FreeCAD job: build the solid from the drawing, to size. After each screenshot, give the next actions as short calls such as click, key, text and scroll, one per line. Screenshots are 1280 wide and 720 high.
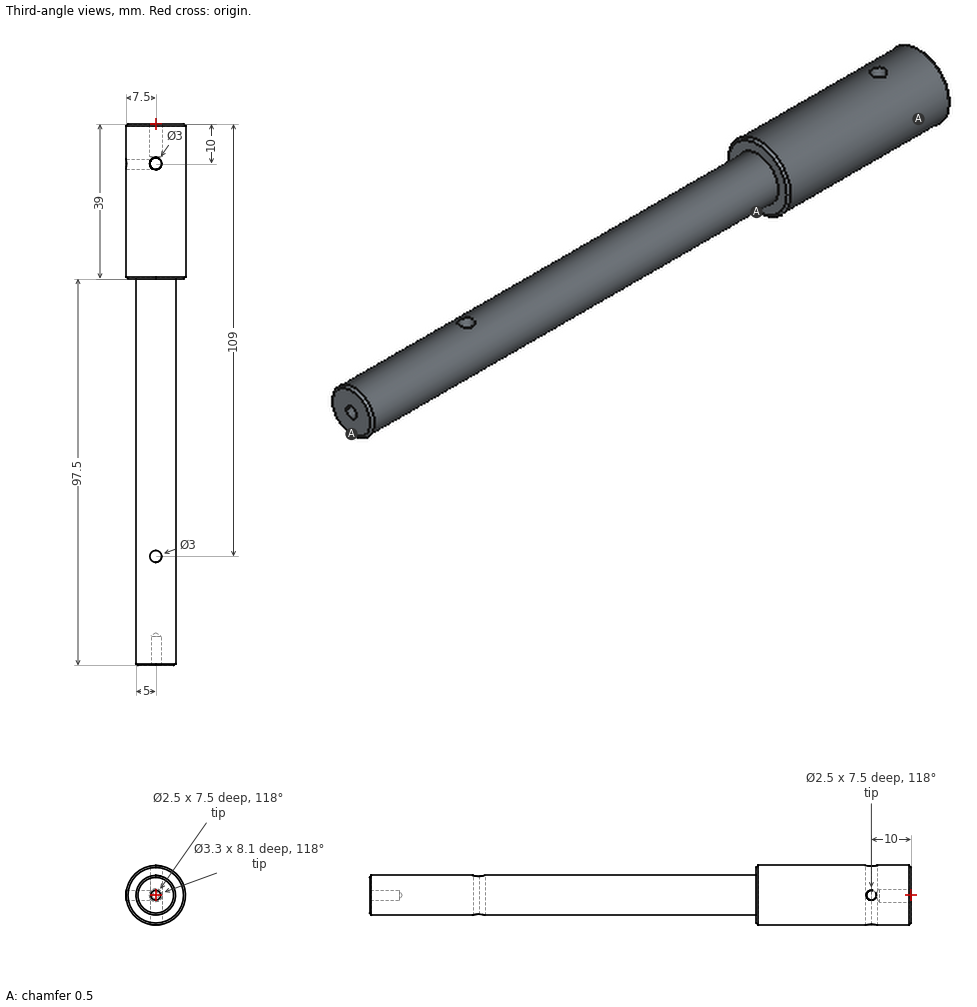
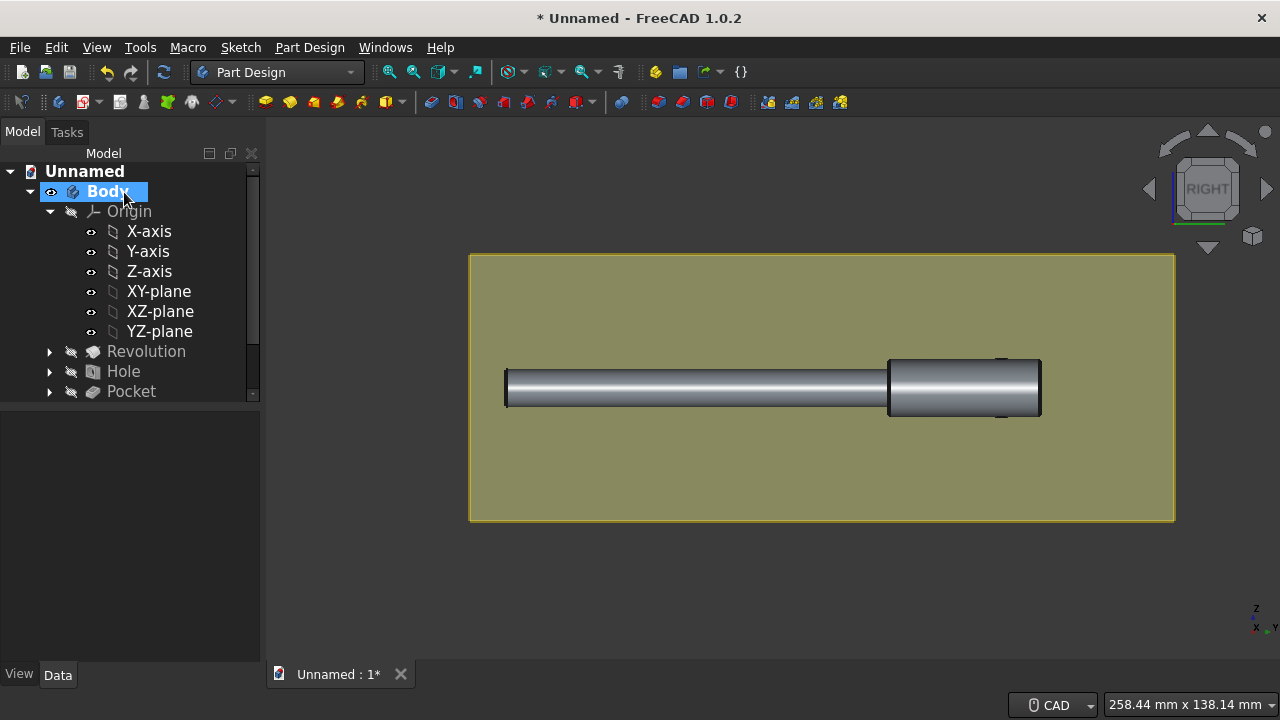
scroll(100, 287, down, 3)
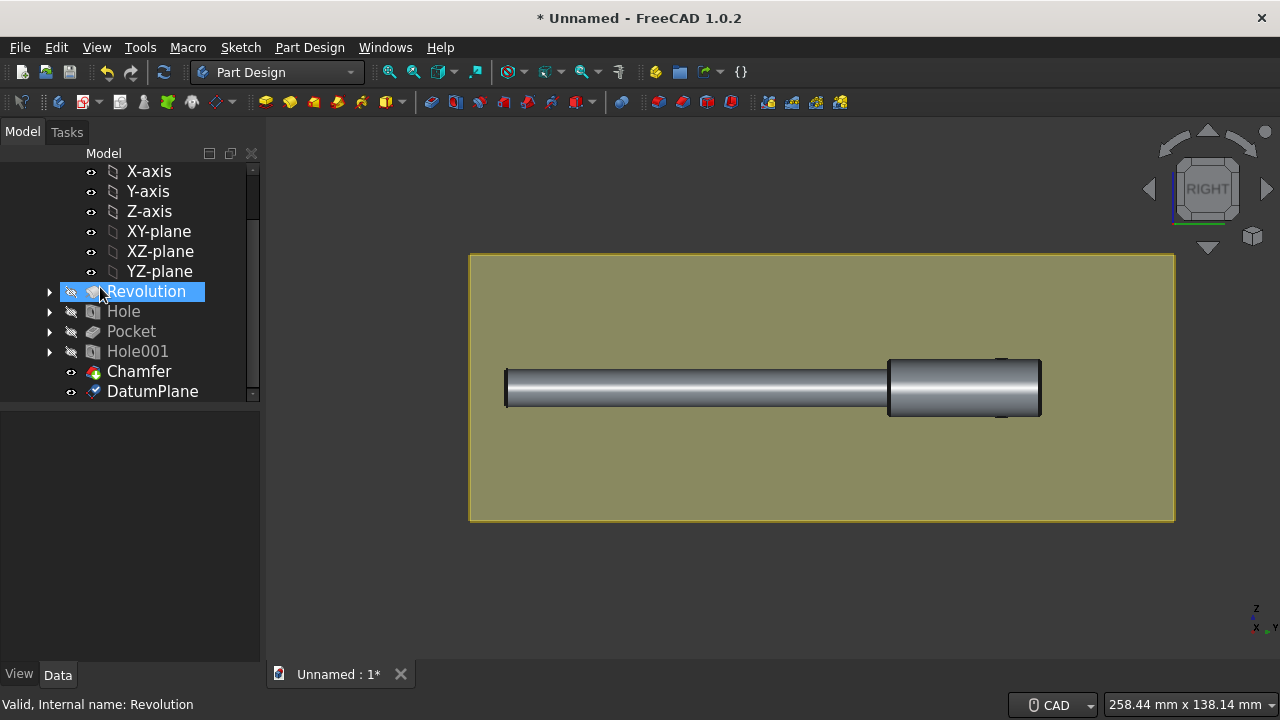
click(116, 392)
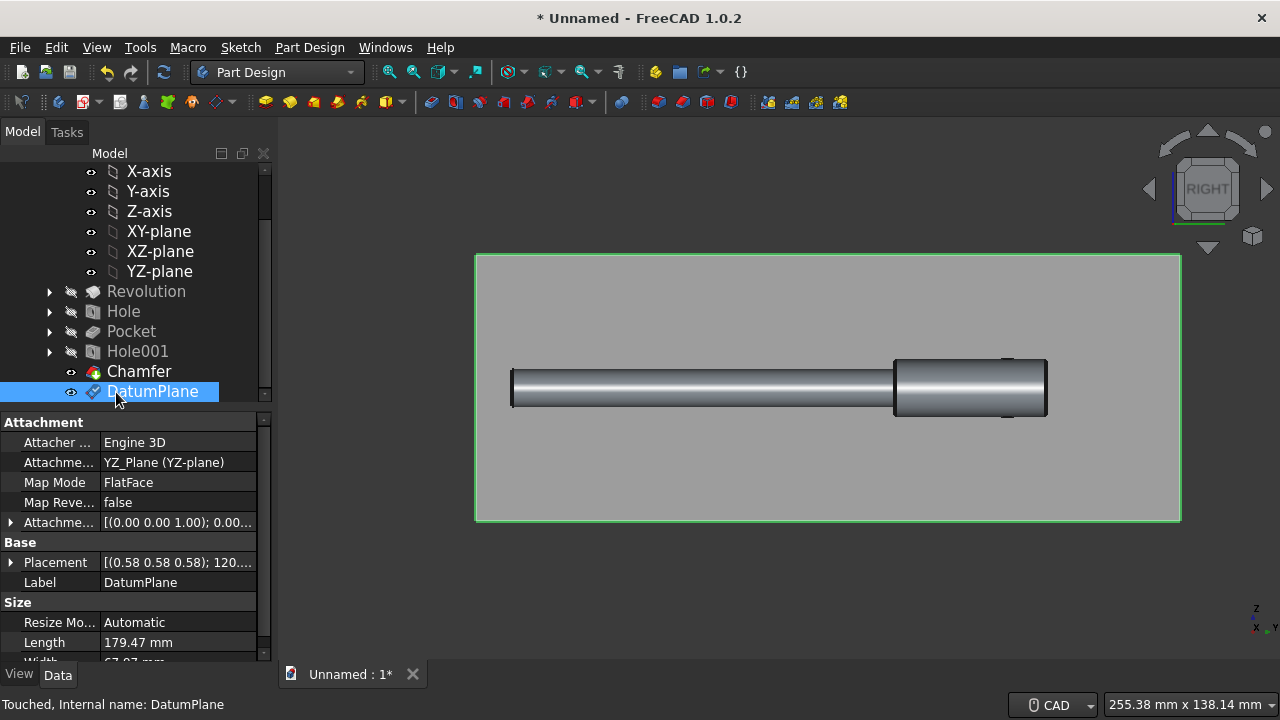
click(84, 102)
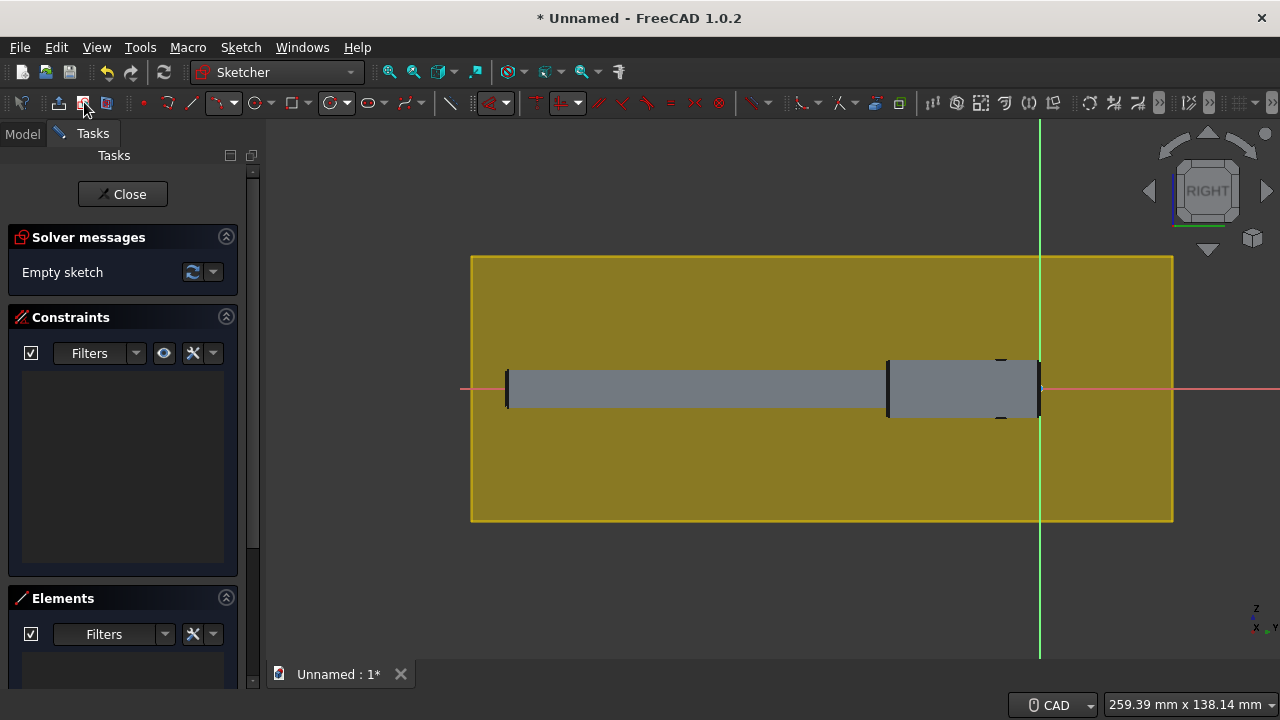
click(108, 104)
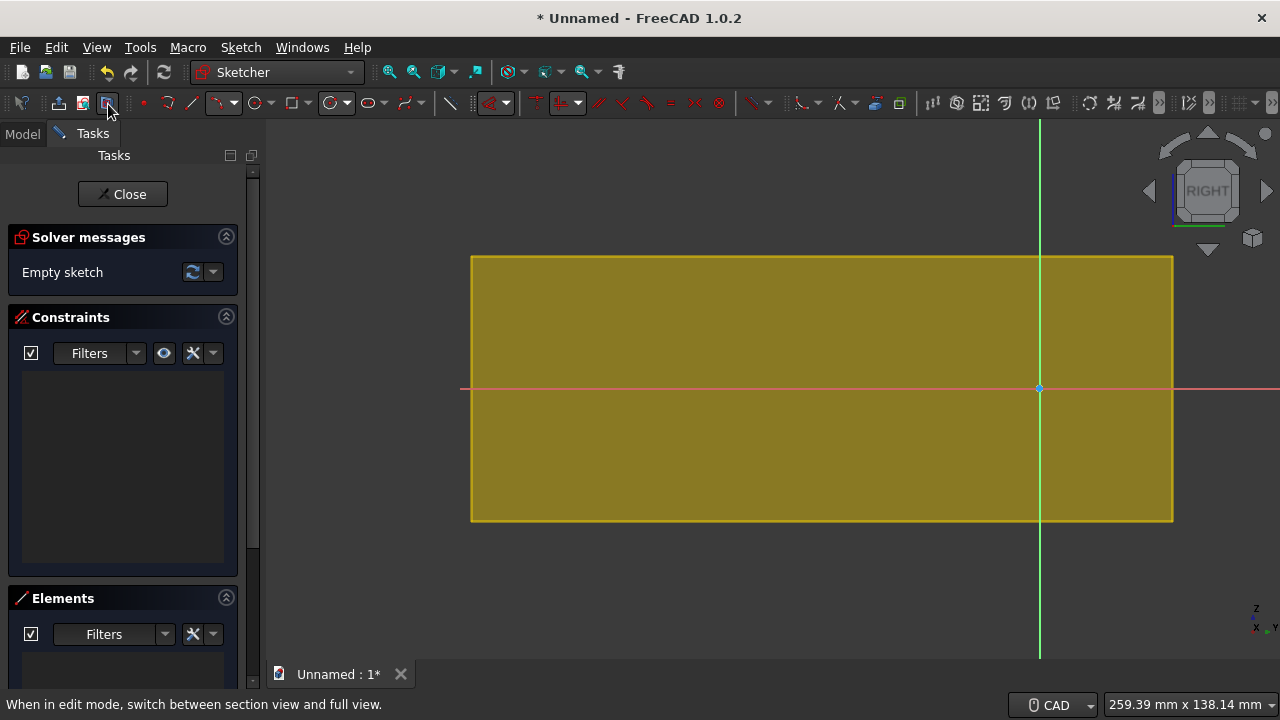
scroll(1016, 389, up, 15)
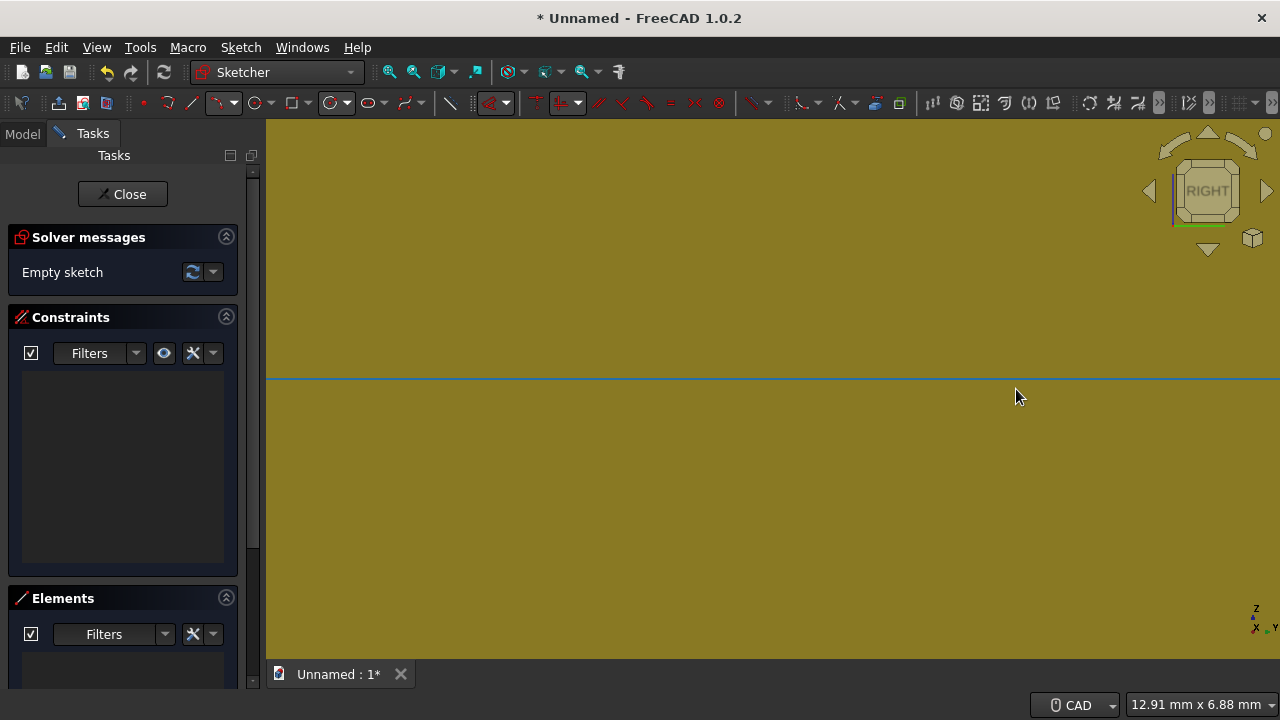
scroll(683, 368, up, 3)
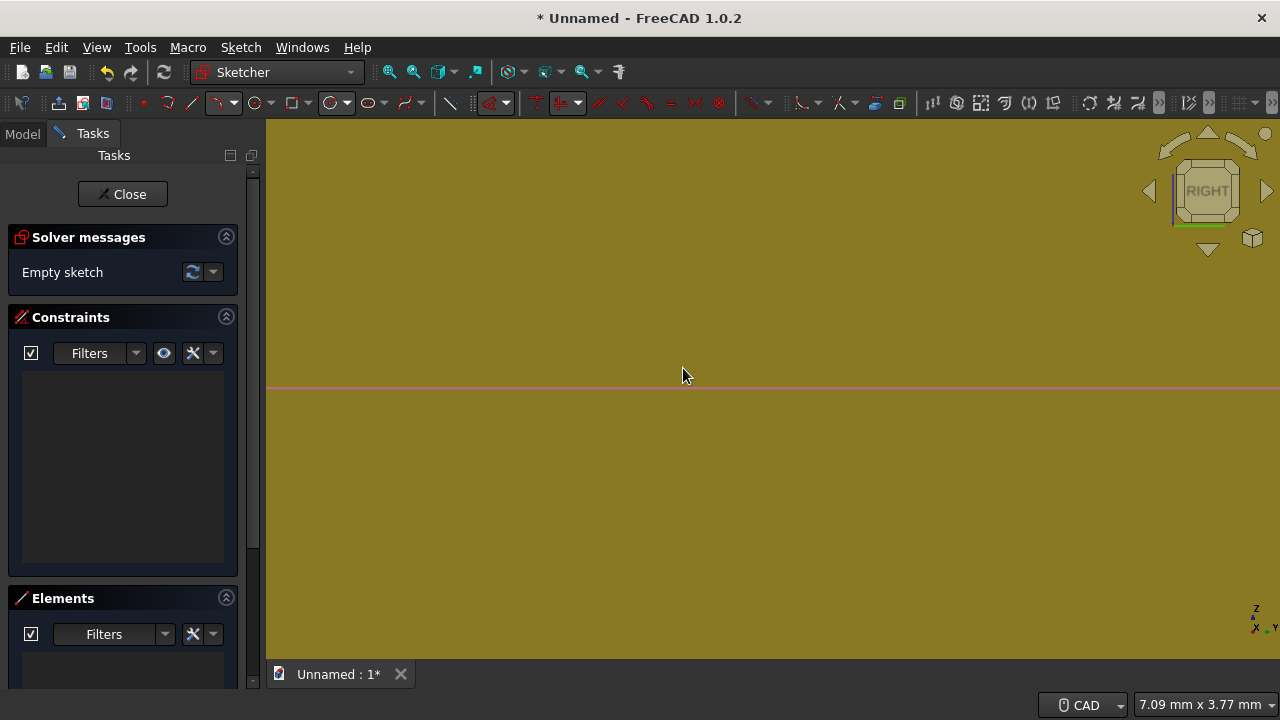
click(256, 104)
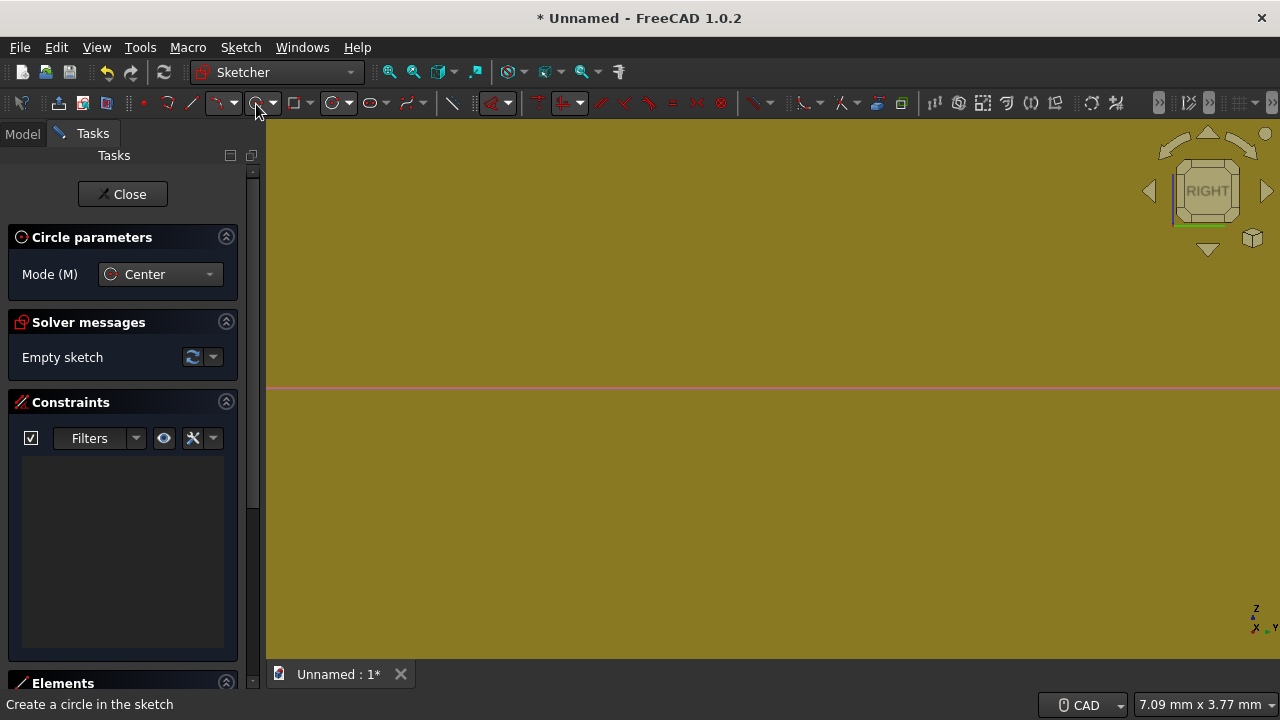
click(704, 388)
click(830, 262)
key(Escape)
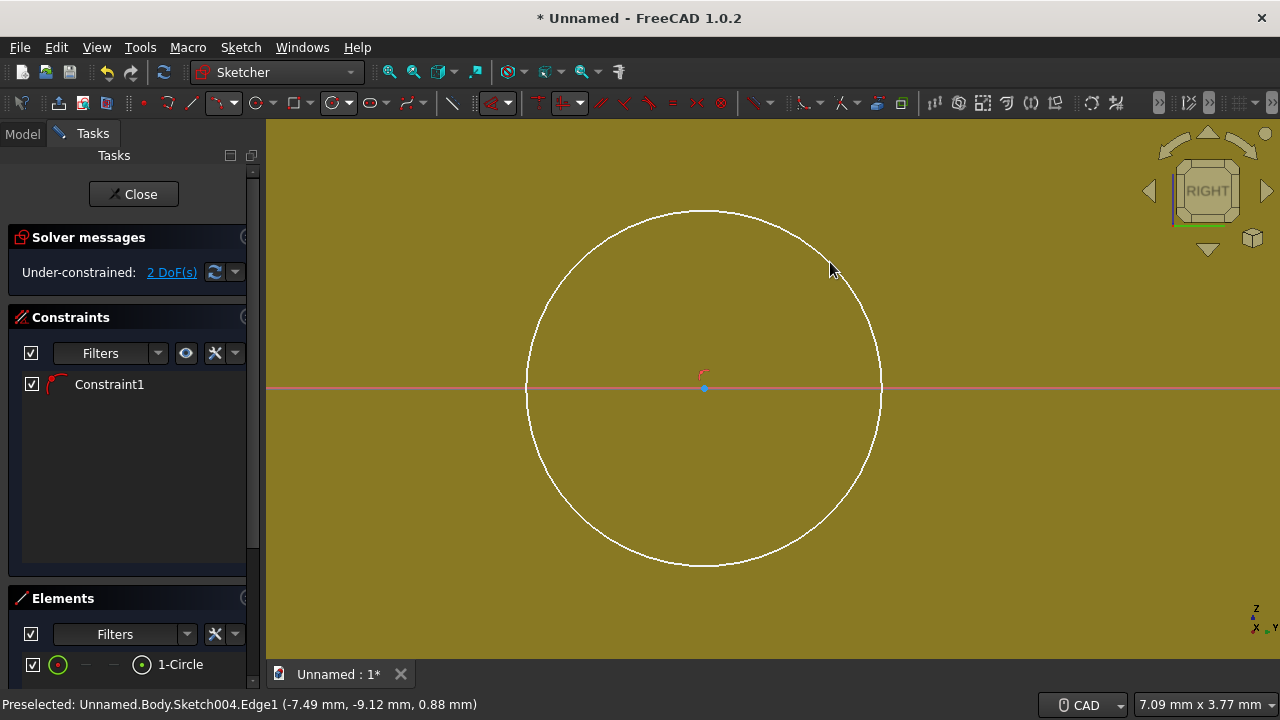
click(829, 262)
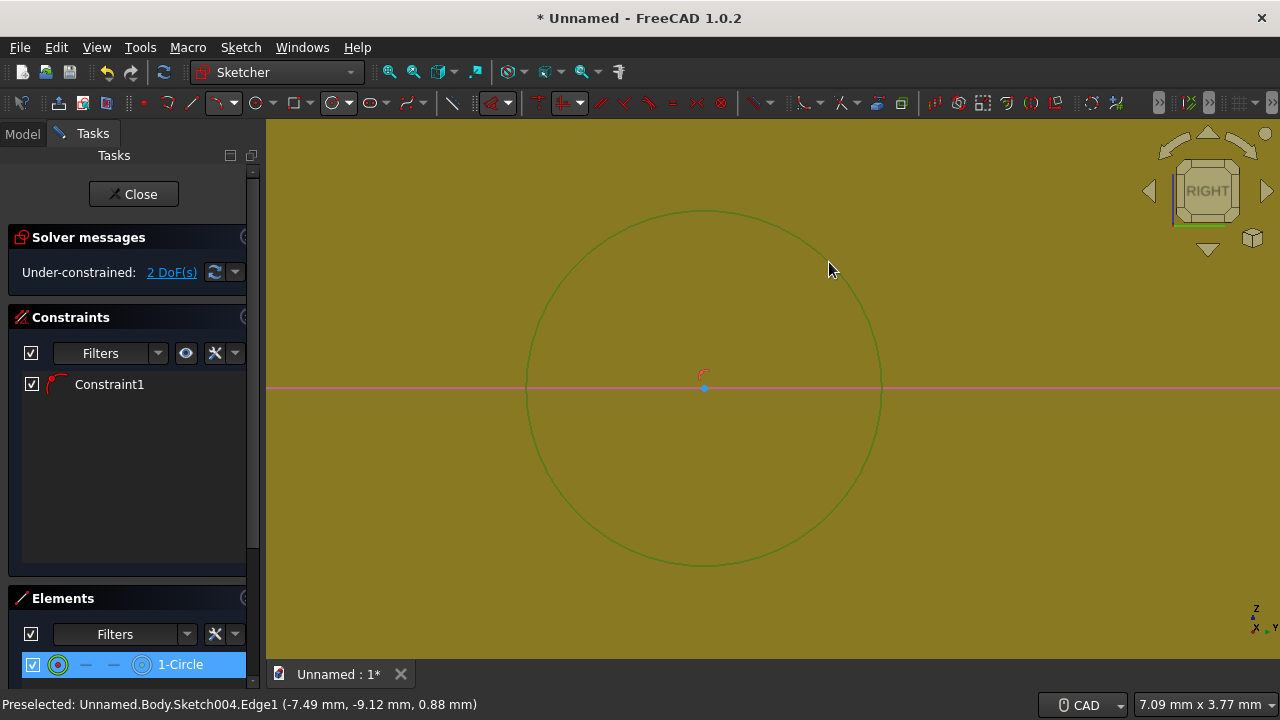
click(510, 104)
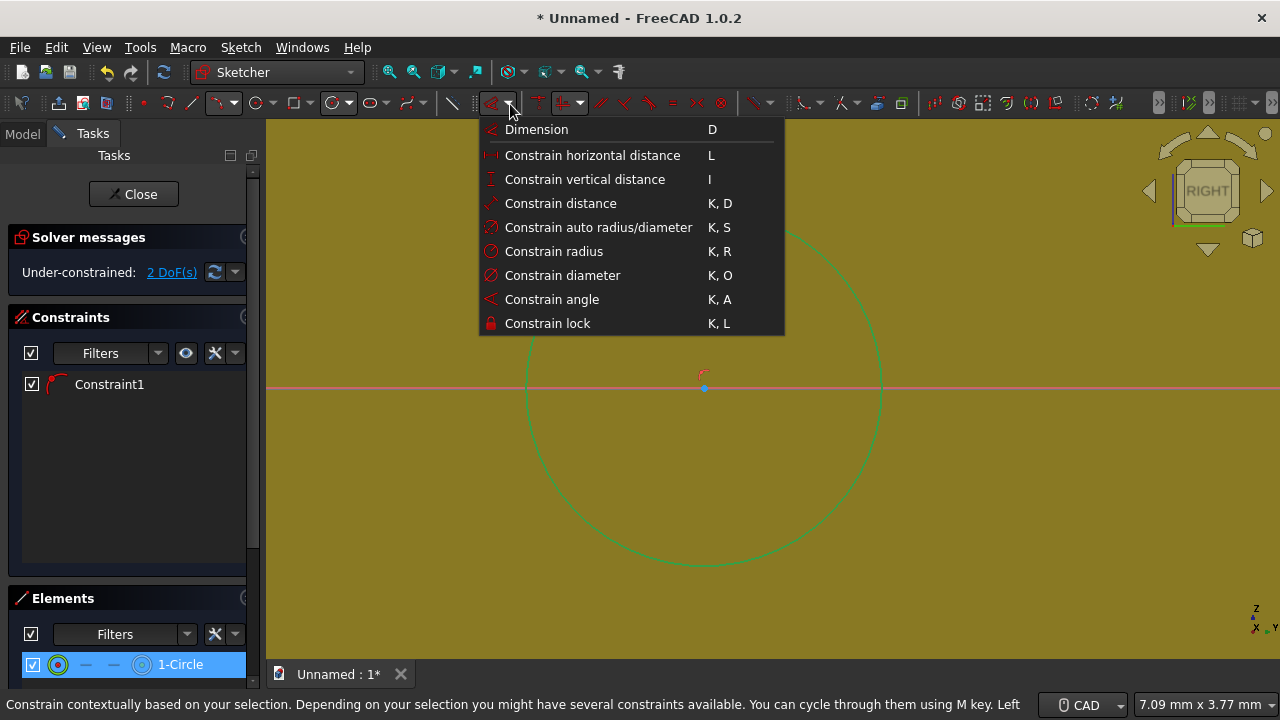
click(632, 275)